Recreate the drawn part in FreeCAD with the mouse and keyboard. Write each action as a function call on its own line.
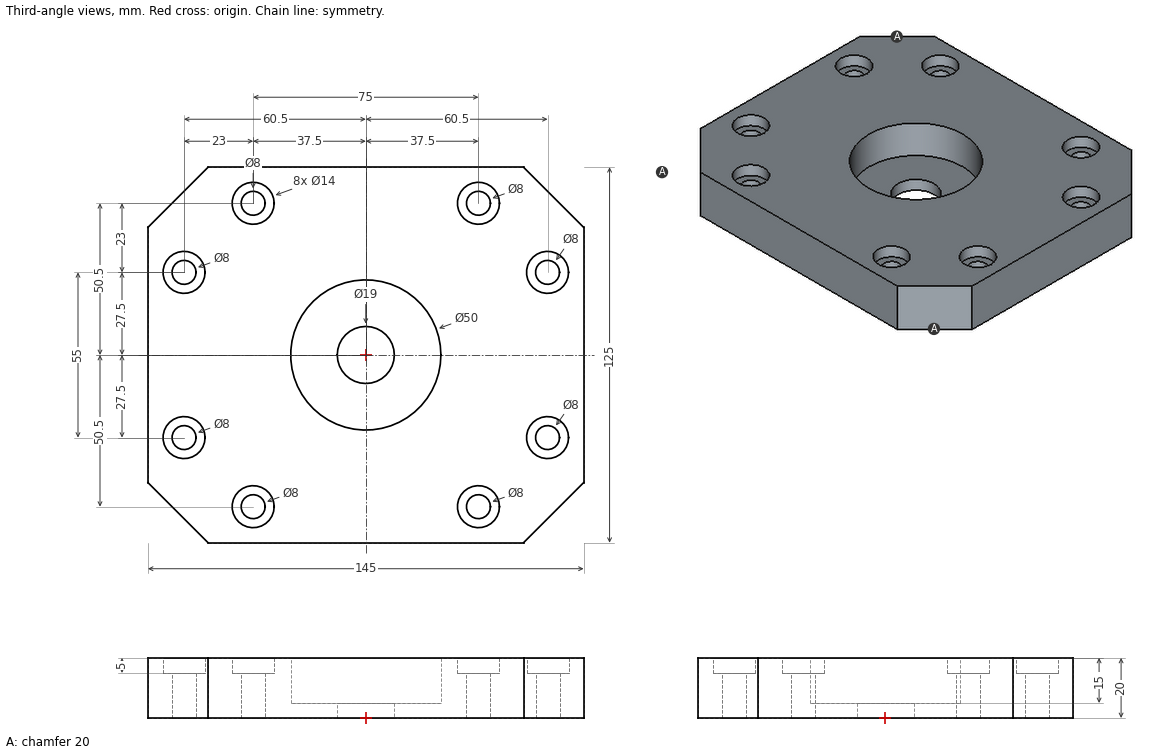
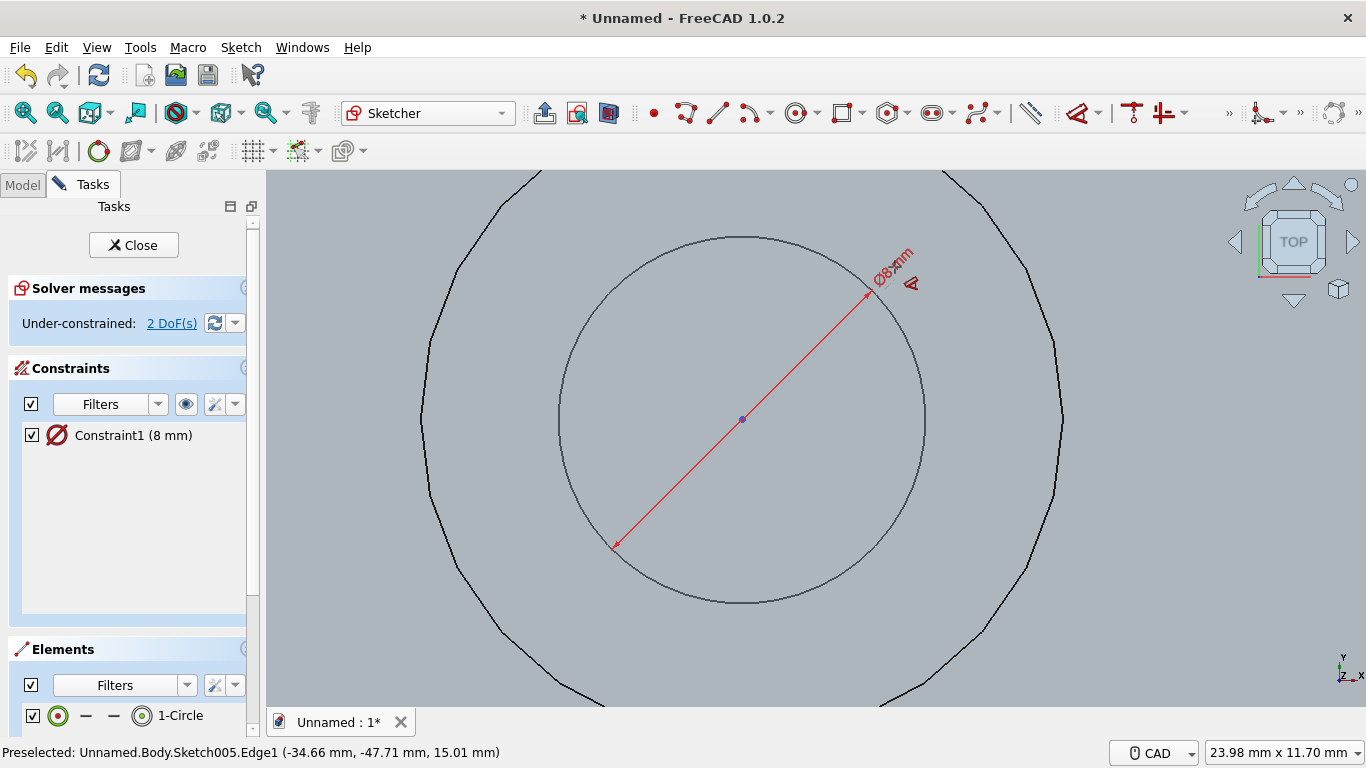
click(742, 420)
click(972, 454)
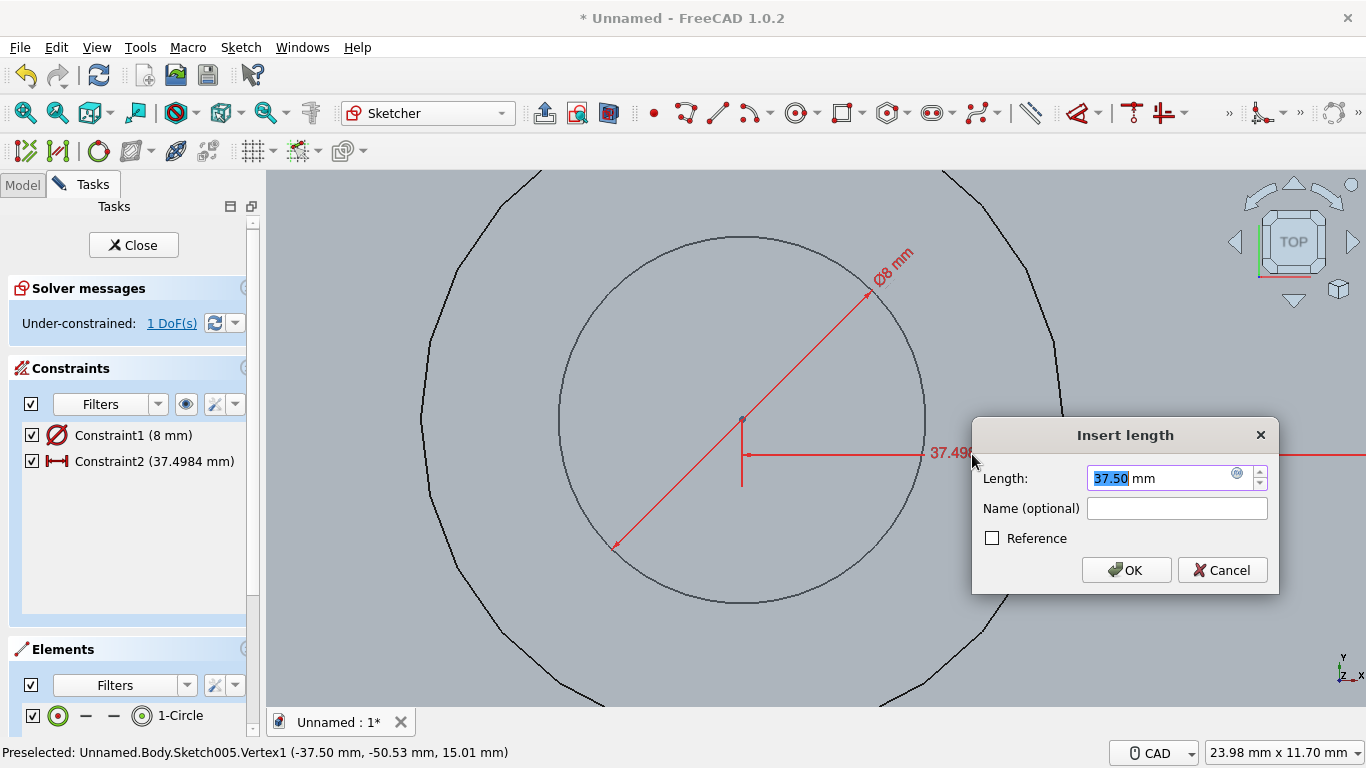
text(37.5)
key(Return)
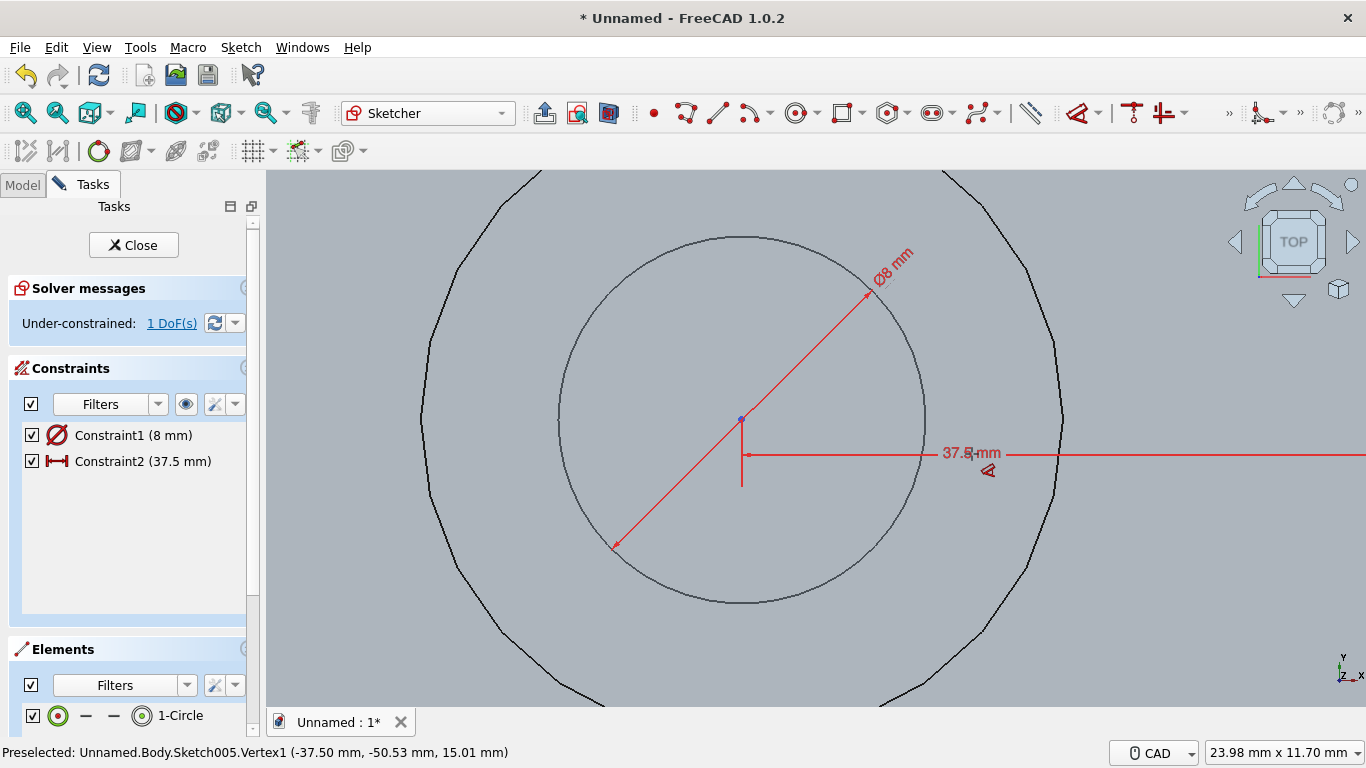
click(742, 420)
click(708, 309)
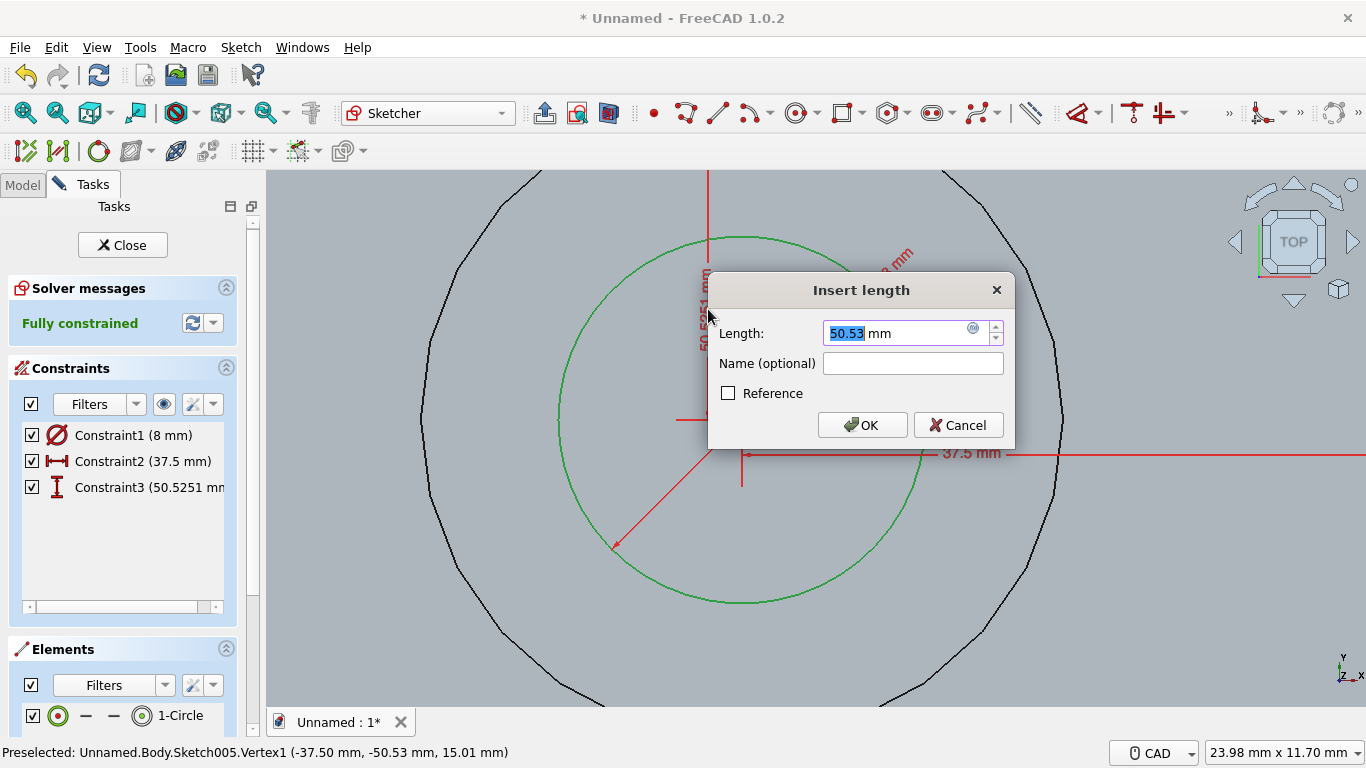
text(50.5)
key(Return)
key(Escape)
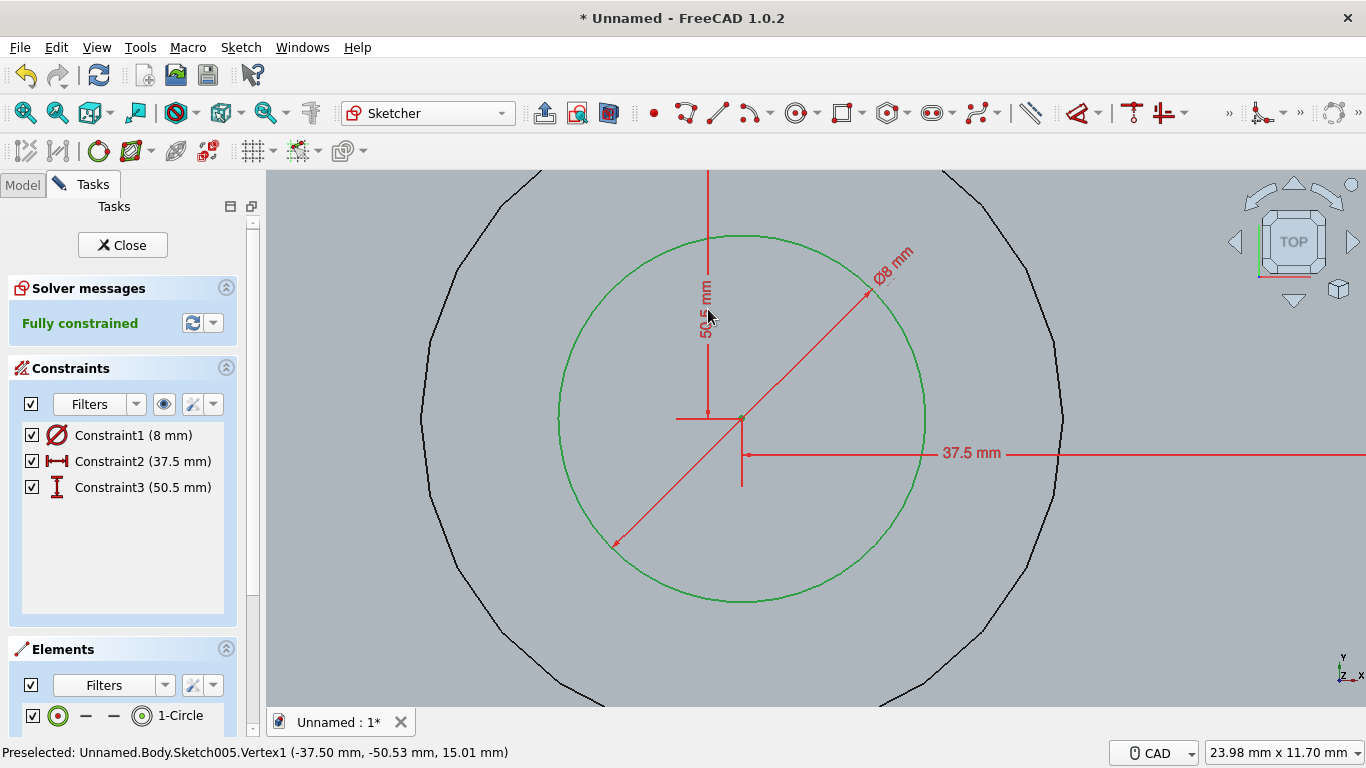
click(123, 245)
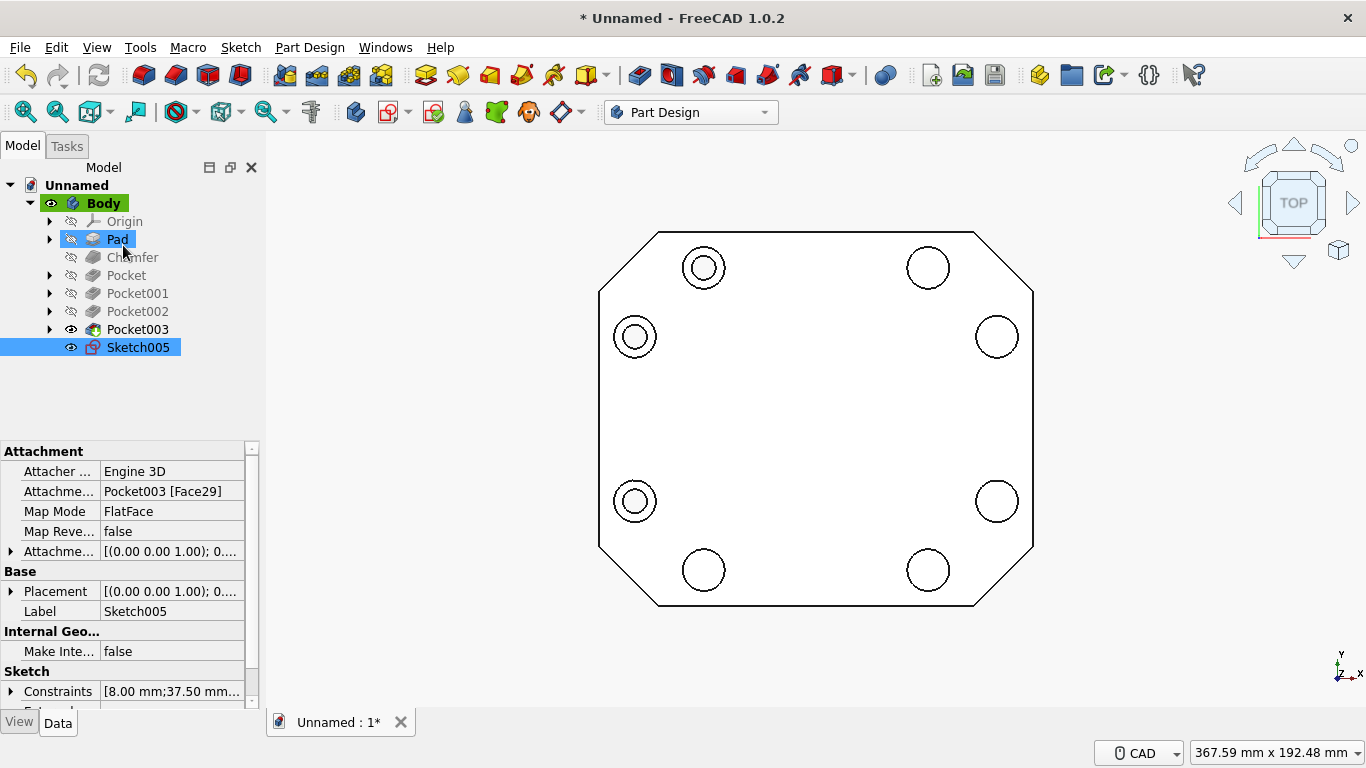
click(640, 76)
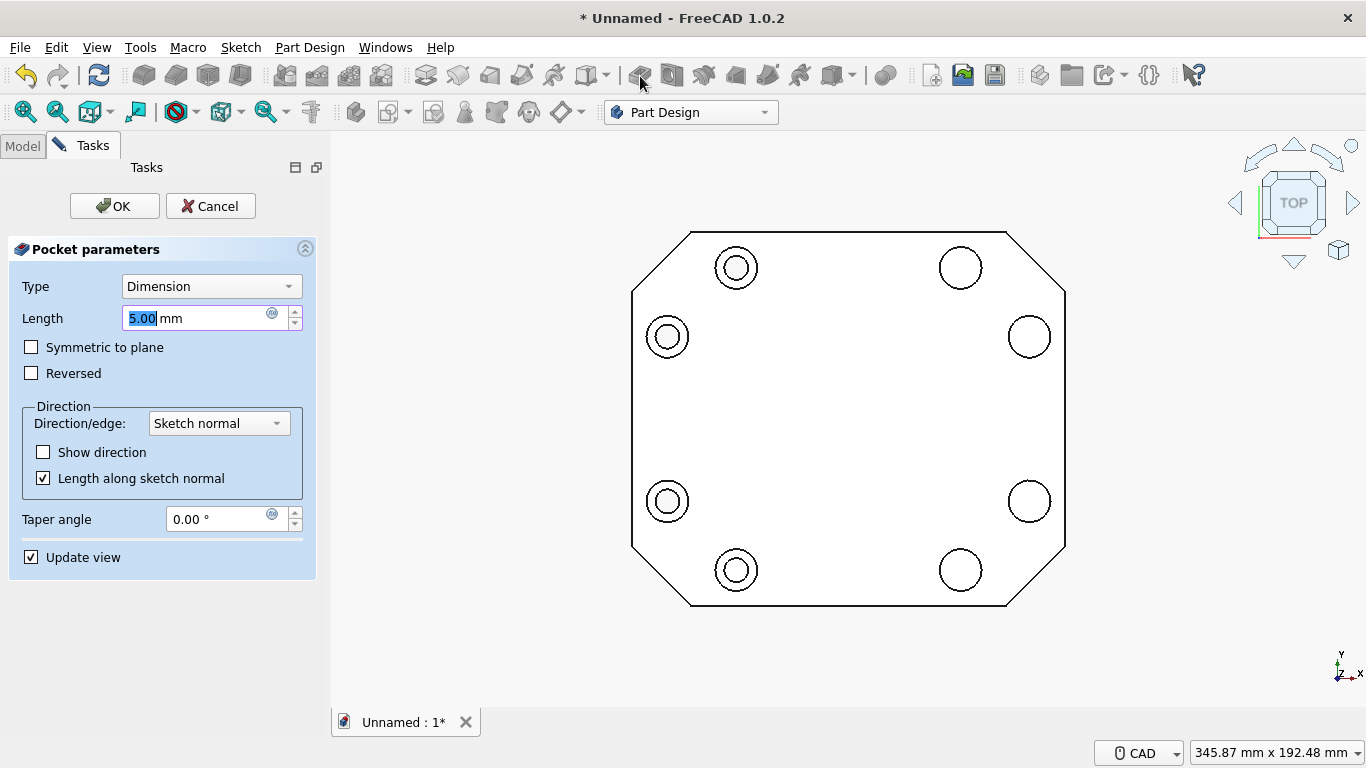
click(212, 286)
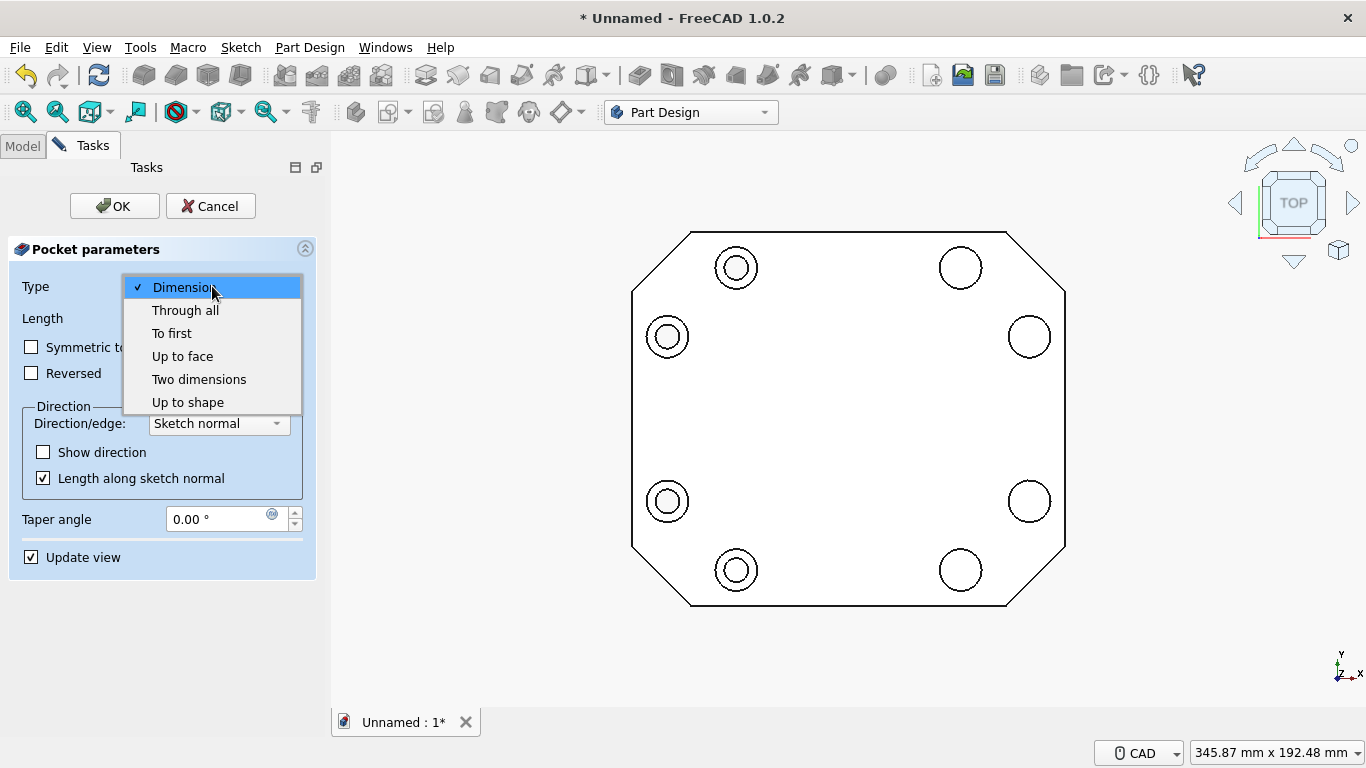
click(212, 334)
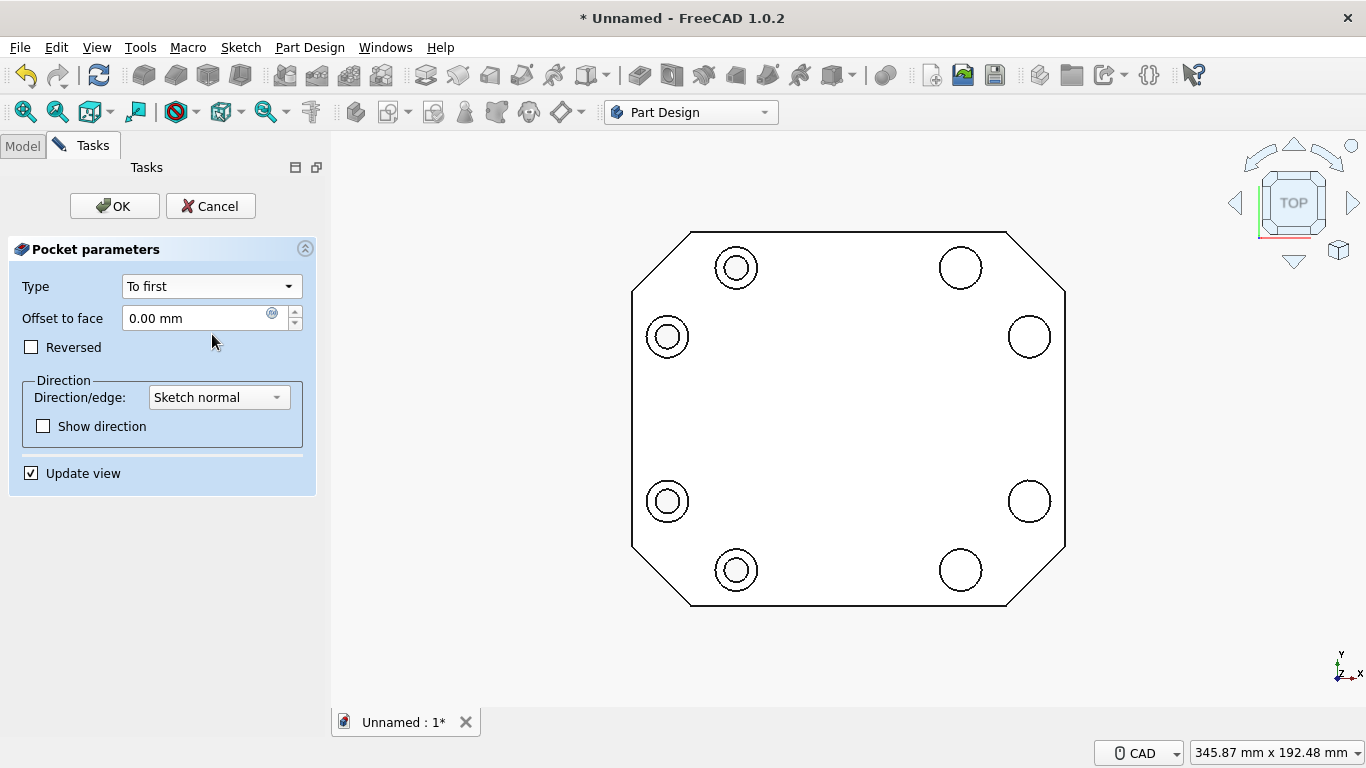
click(115, 206)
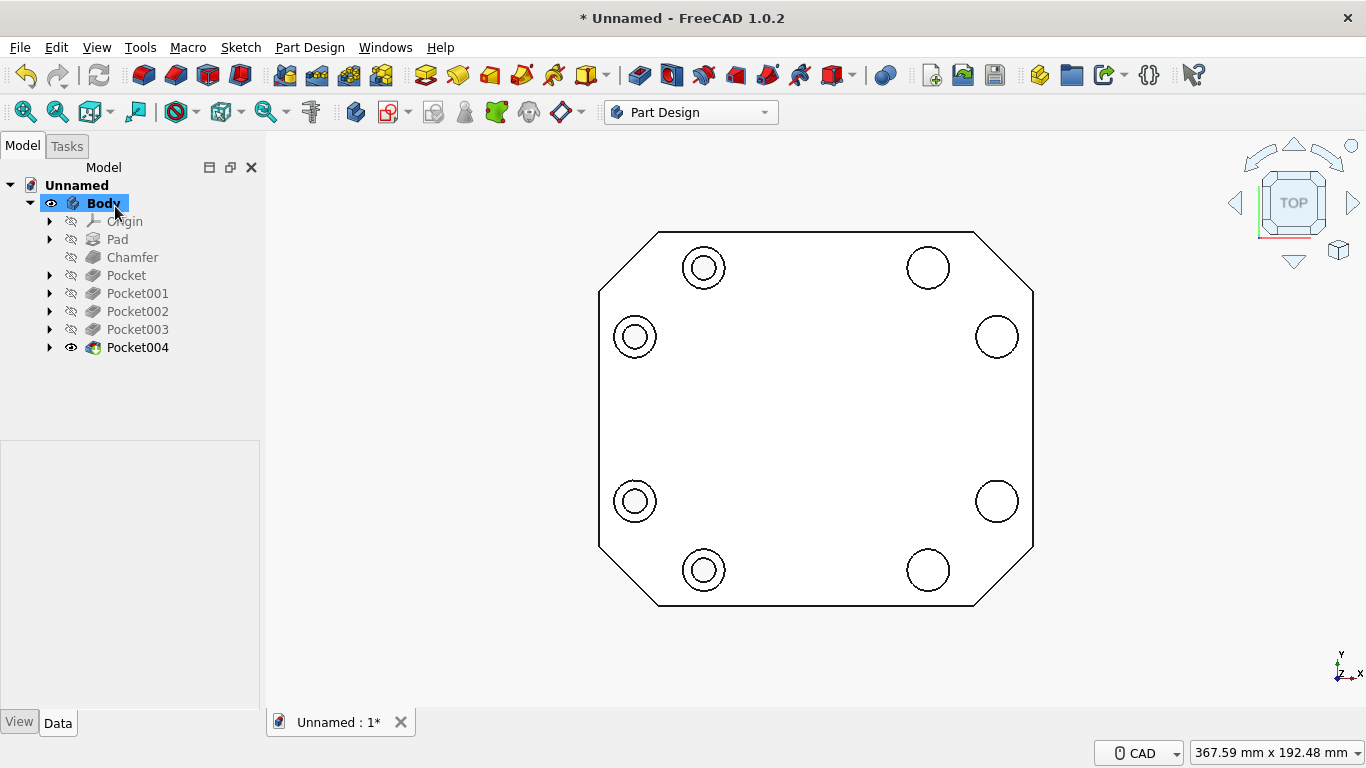
click(928, 267)